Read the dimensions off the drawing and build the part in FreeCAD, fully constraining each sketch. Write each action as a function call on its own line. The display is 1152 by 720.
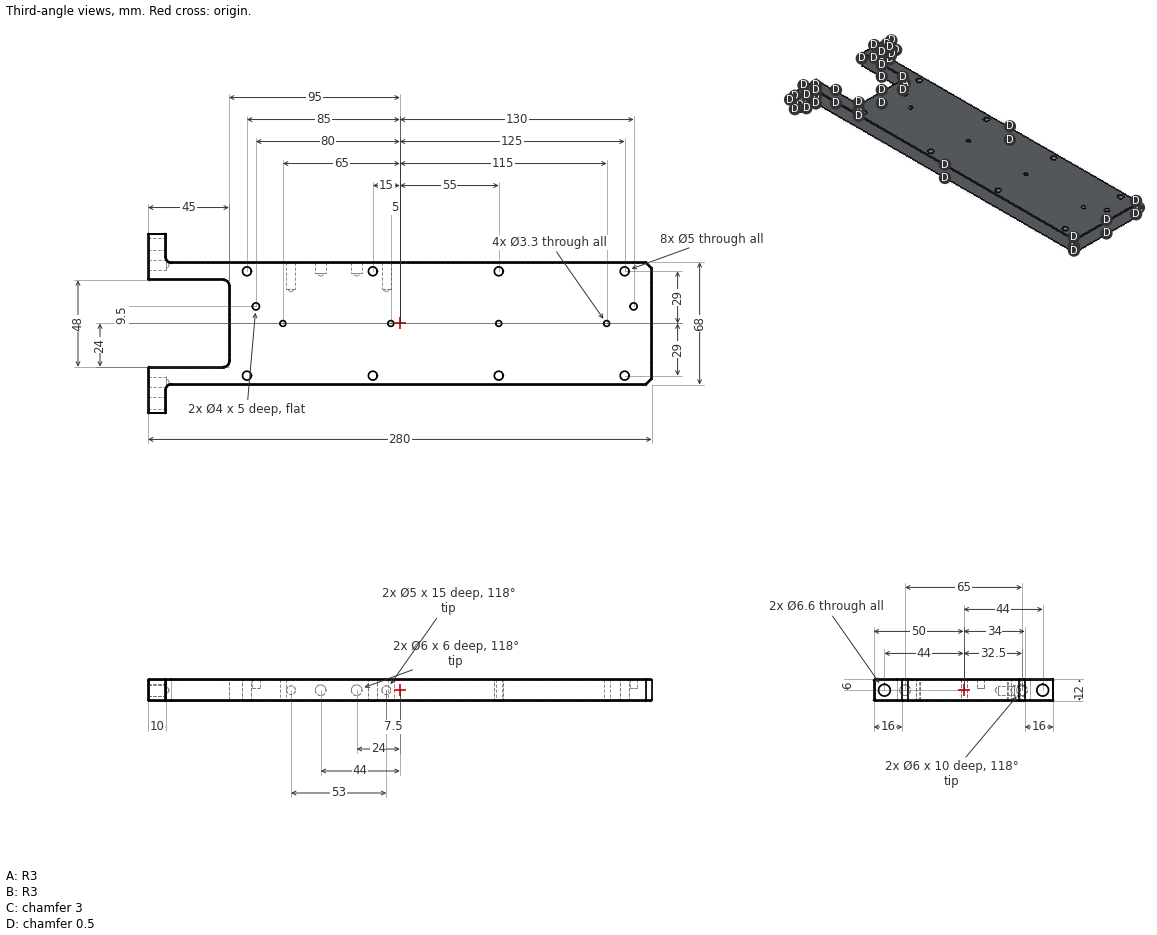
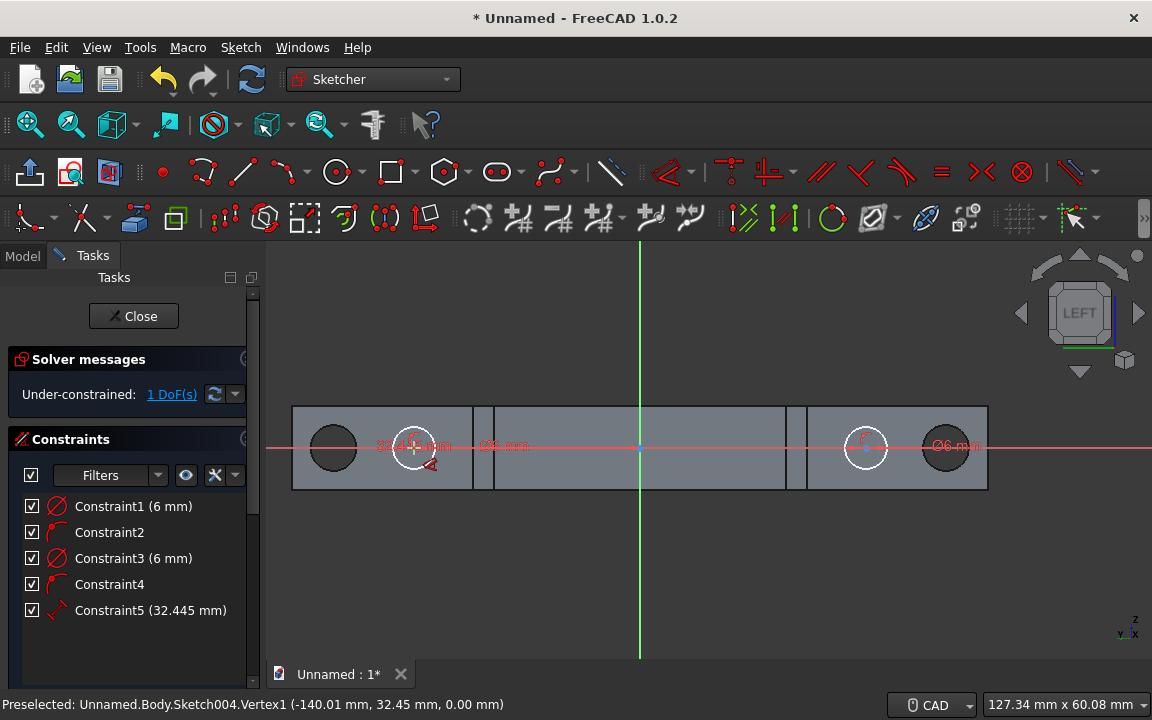
click(866, 448)
click(536, 482)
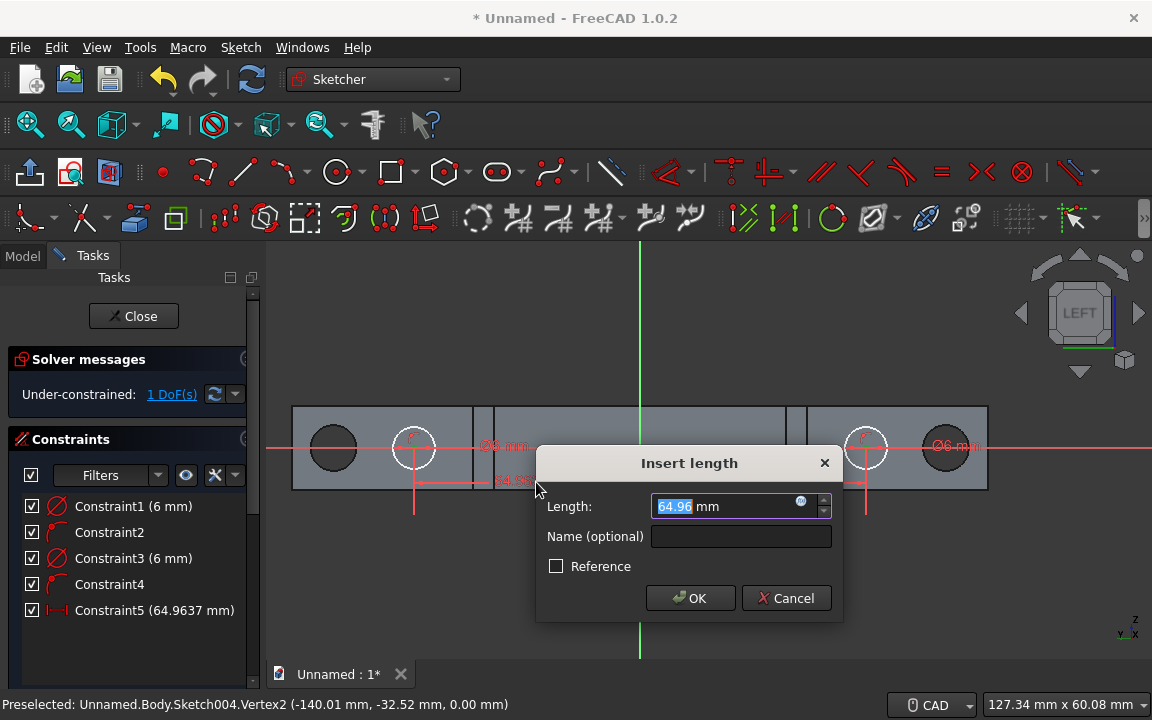
text(65)
key(Return)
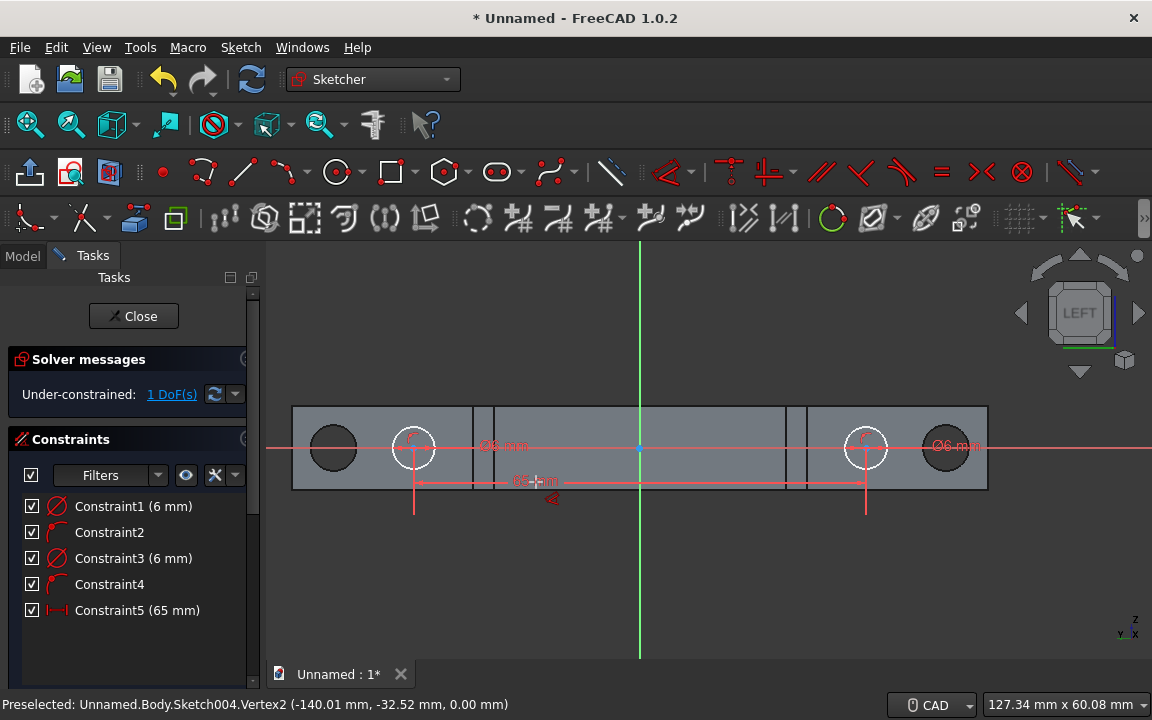
click(414, 448)
click(448, 482)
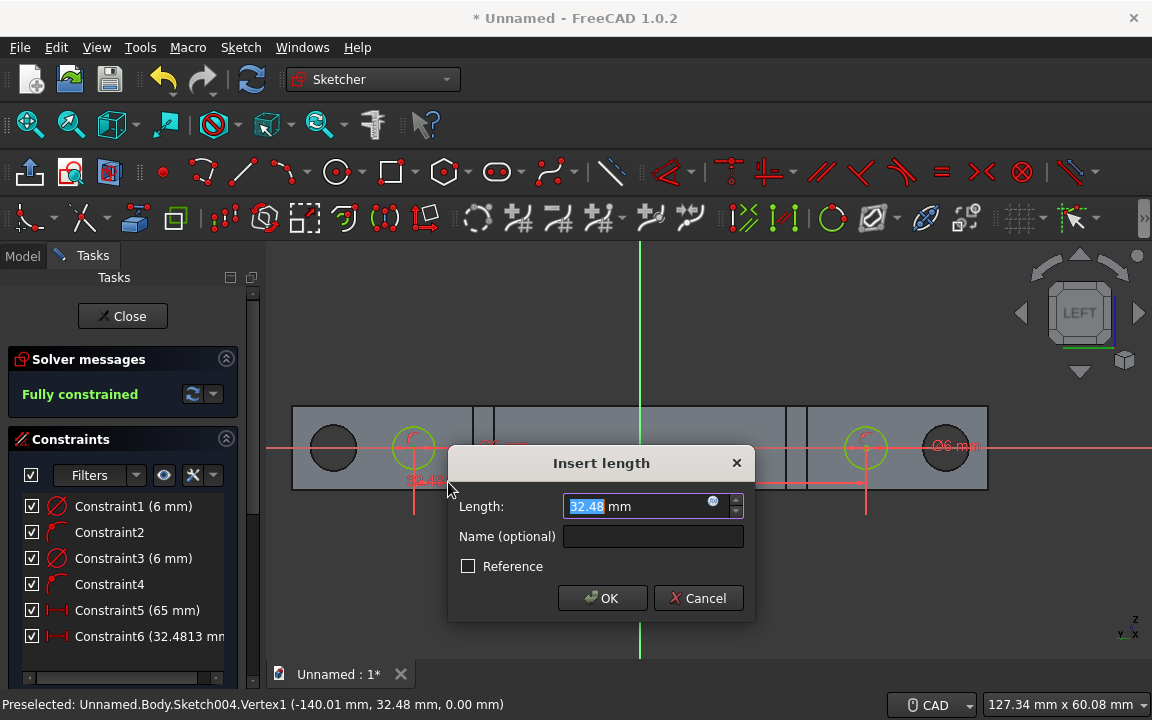
text(32.5)
key(Return)
key(Escape)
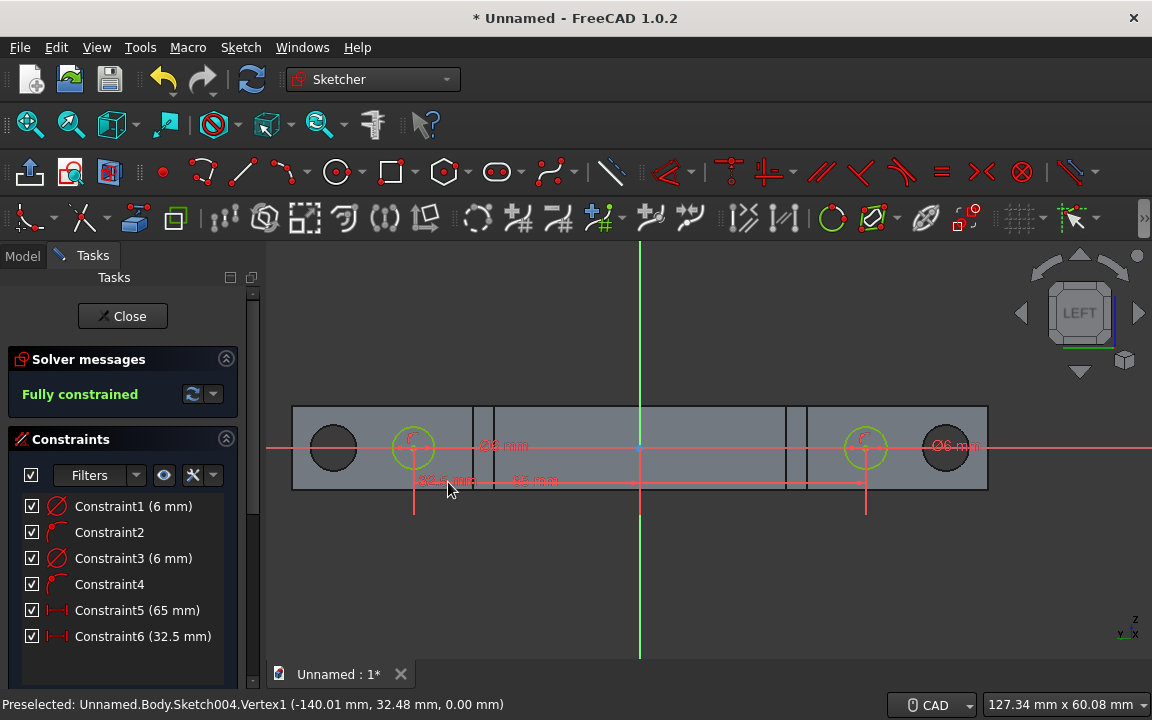
click(123, 316)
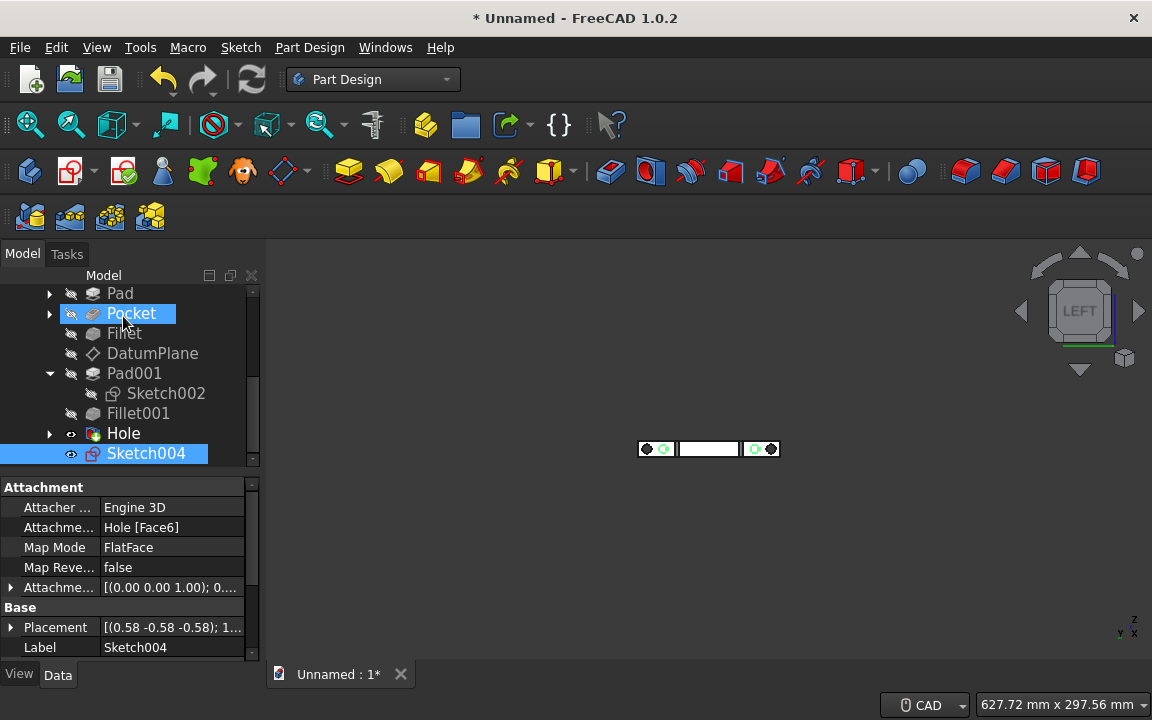
click(652, 172)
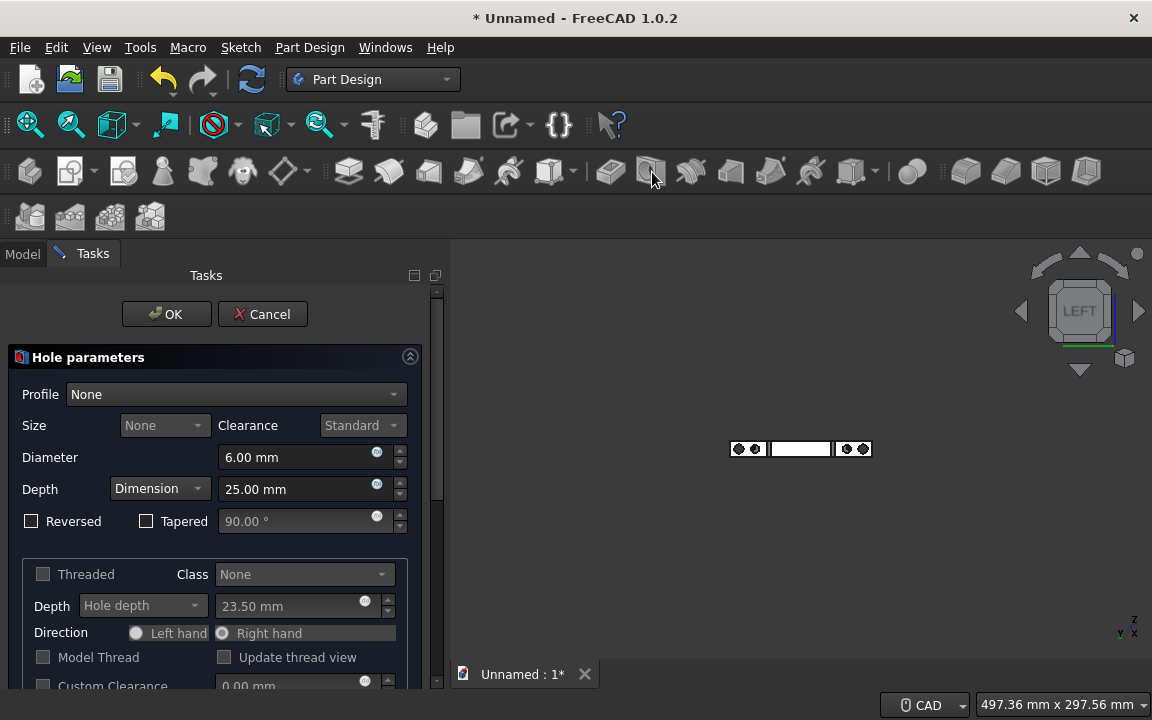
triple_click(305, 457)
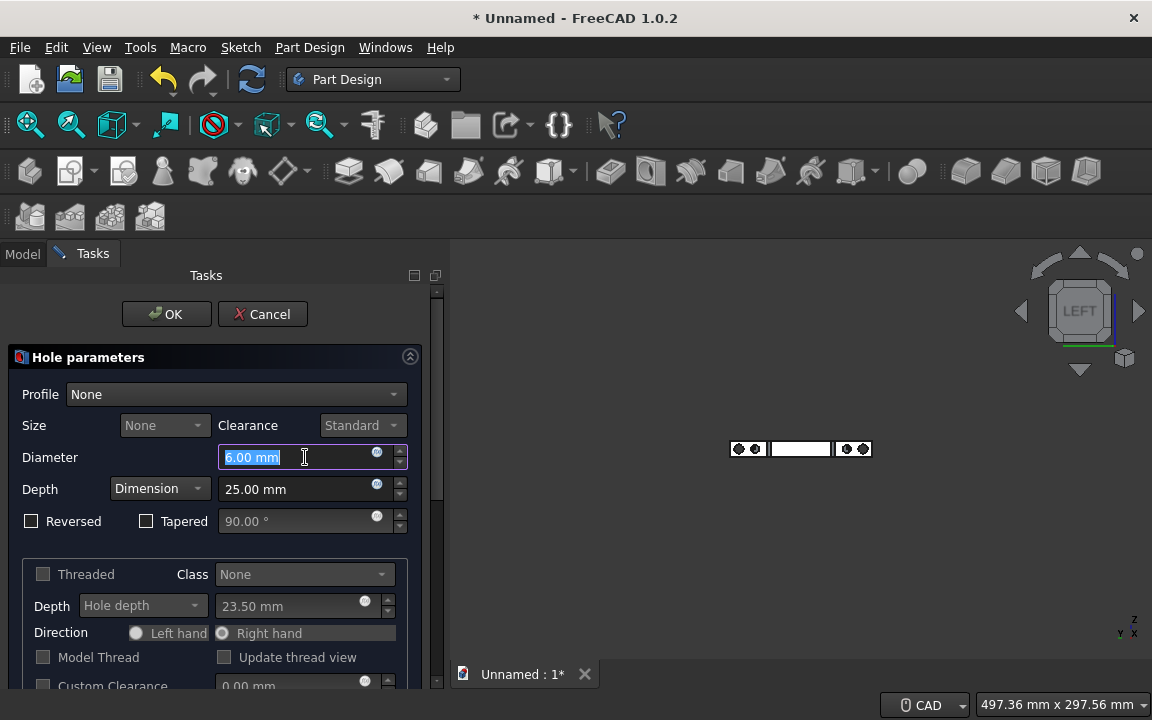
text(6)
key(Tab)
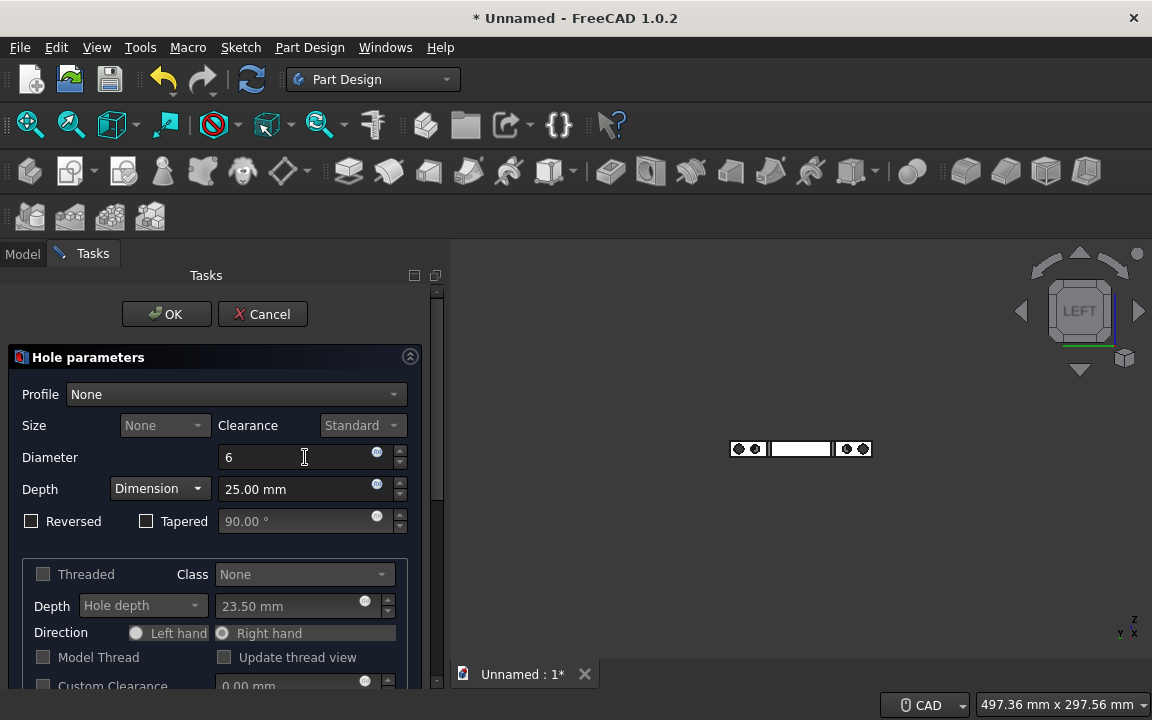
triple_click(305, 489)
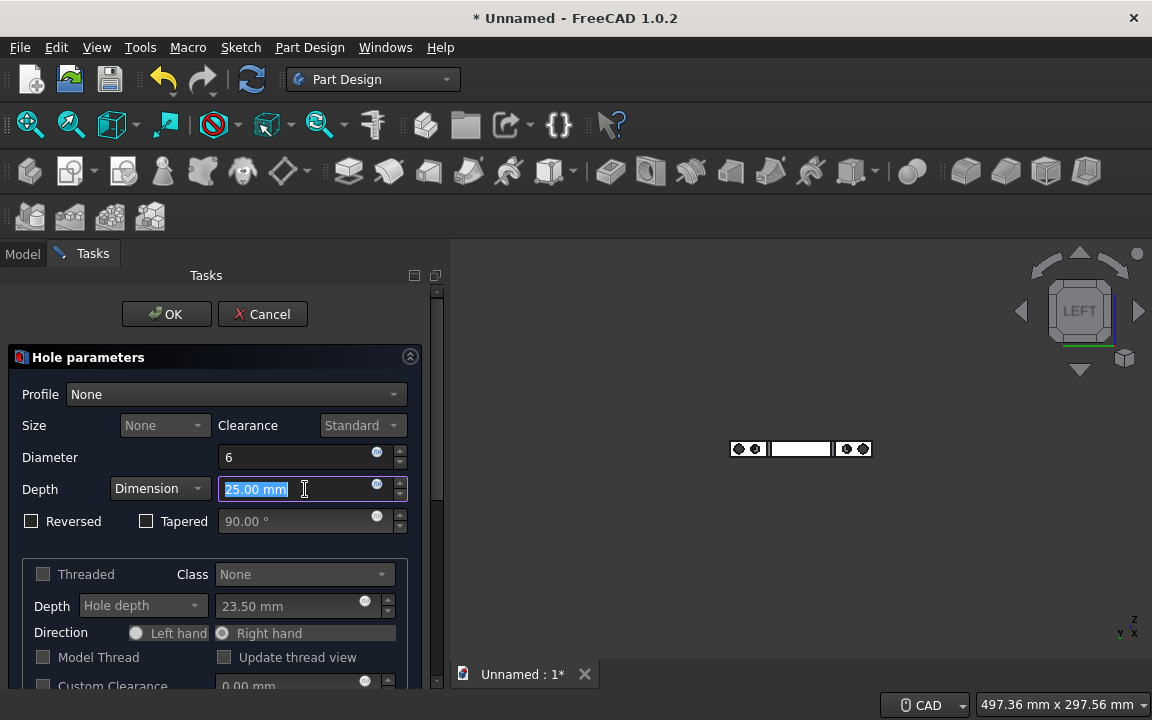
text(10)
key(Tab)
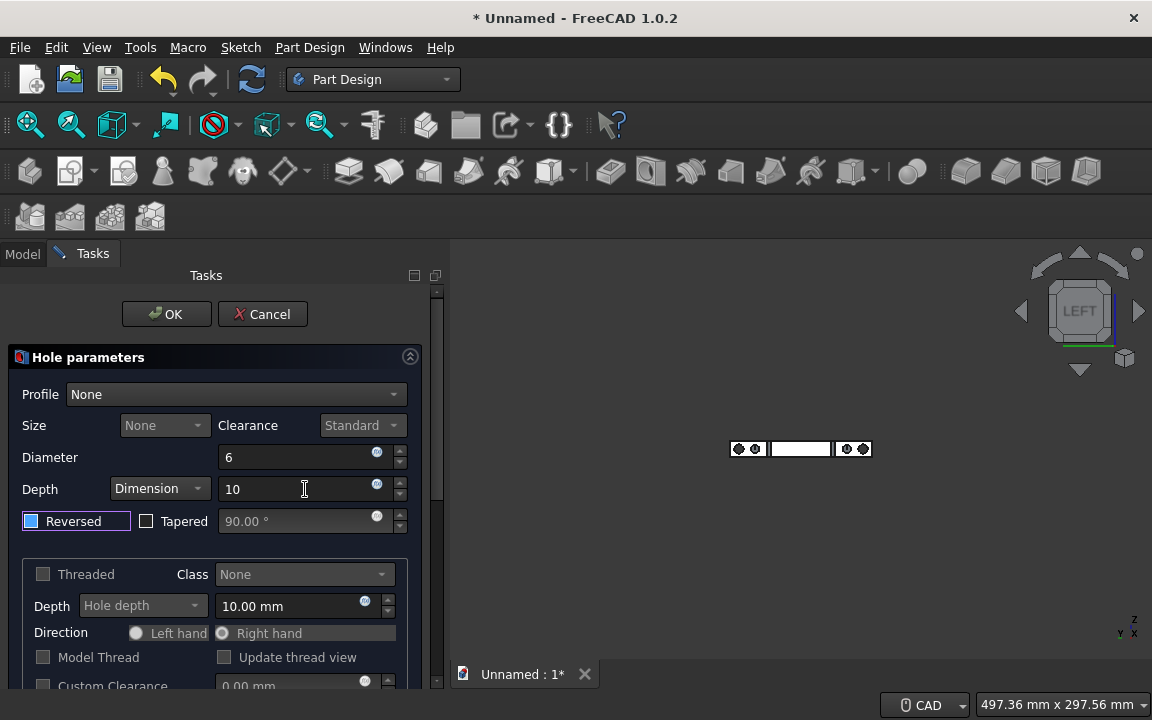
click(167, 314)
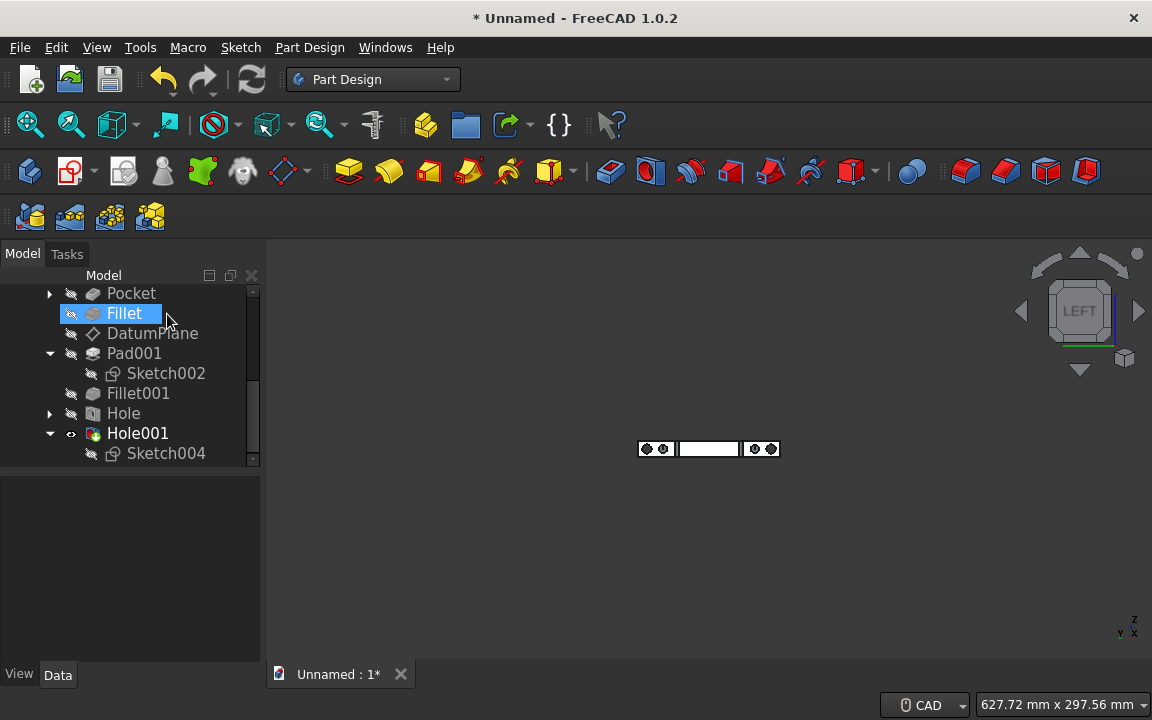
click(32, 126)